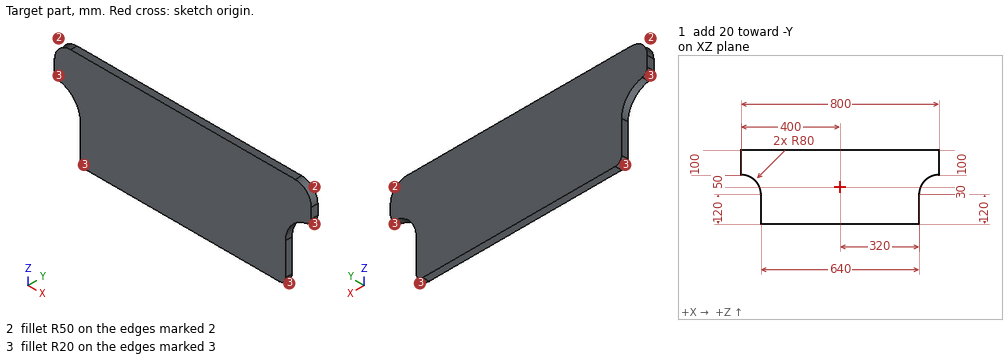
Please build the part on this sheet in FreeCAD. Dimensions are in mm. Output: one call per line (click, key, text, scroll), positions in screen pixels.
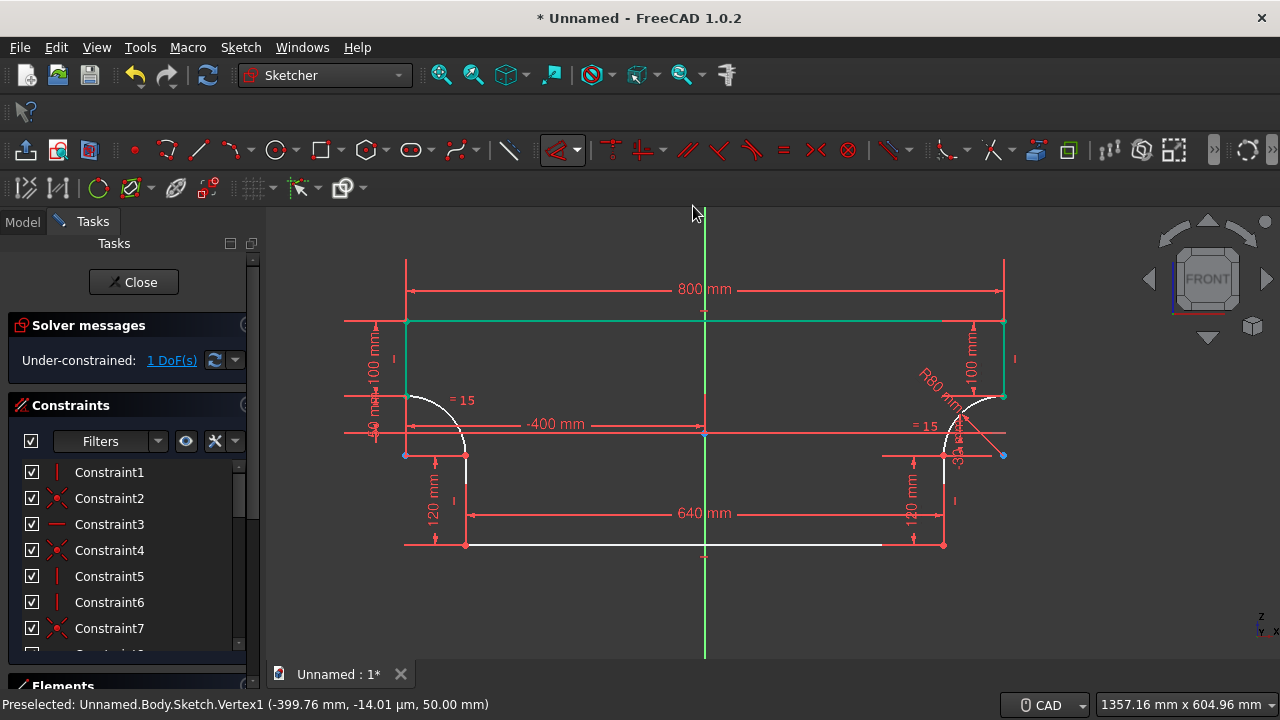
click(944, 456)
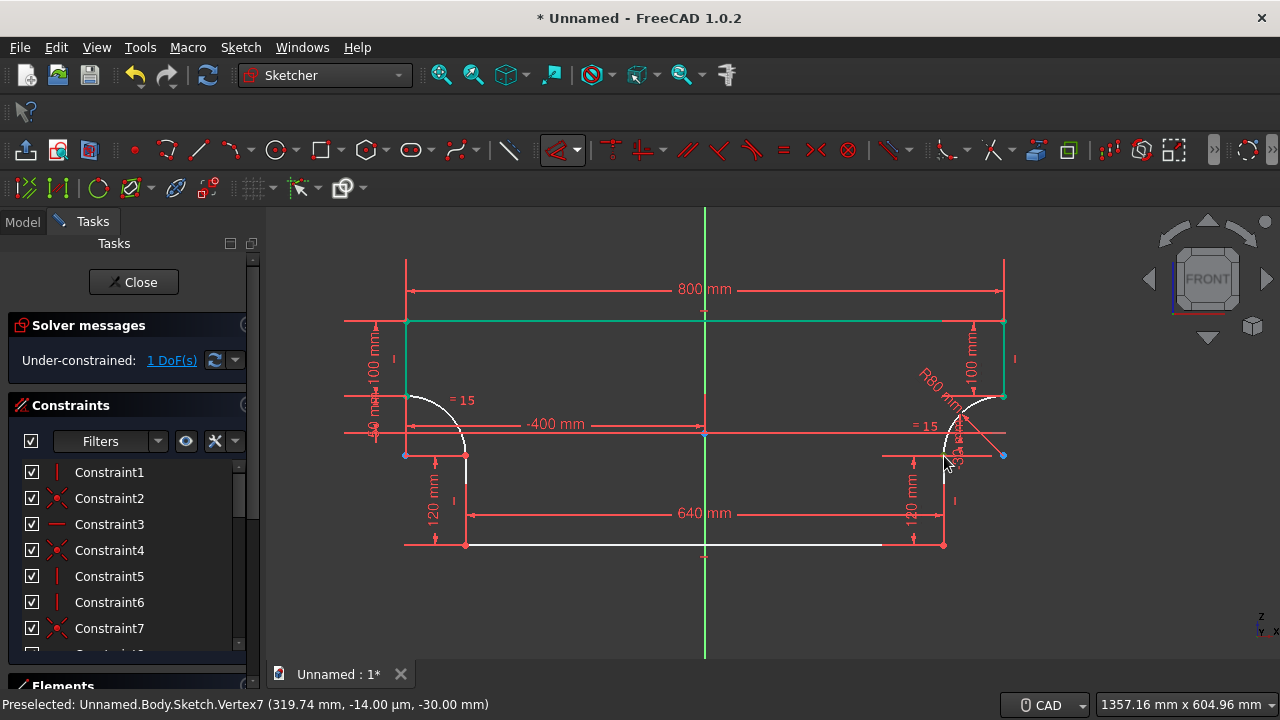
key(l)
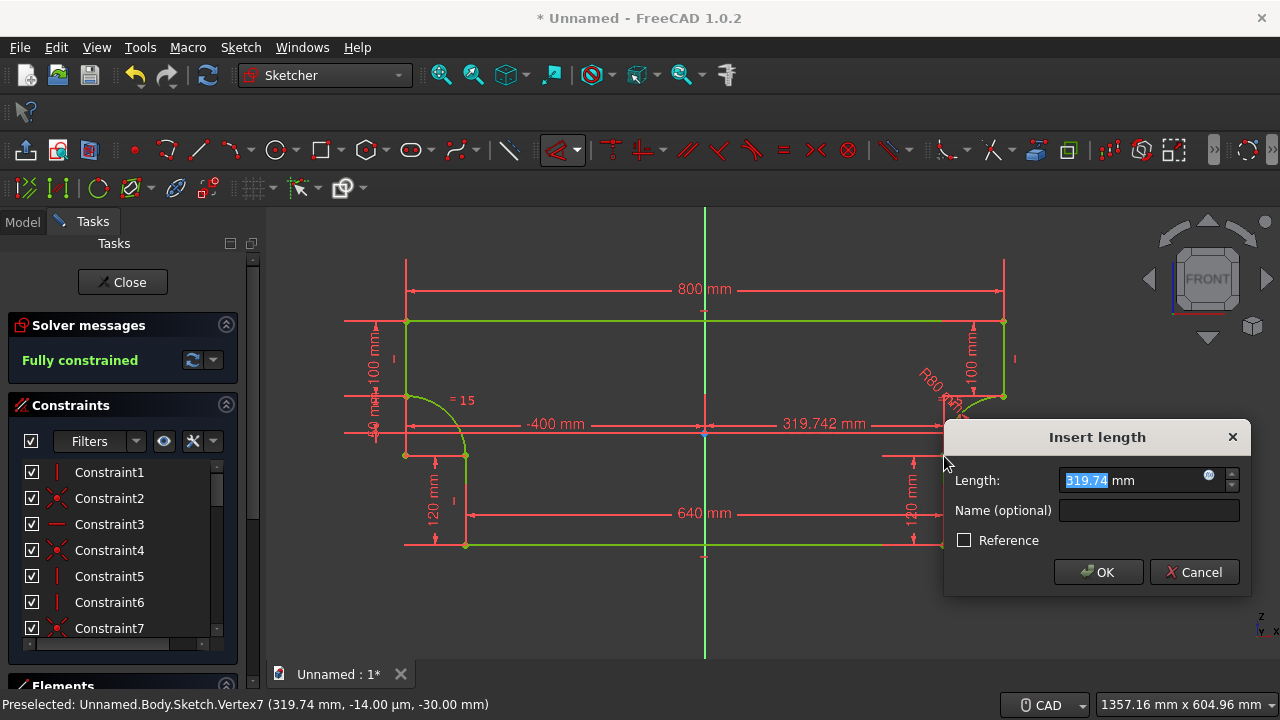
text(320)
key(Return)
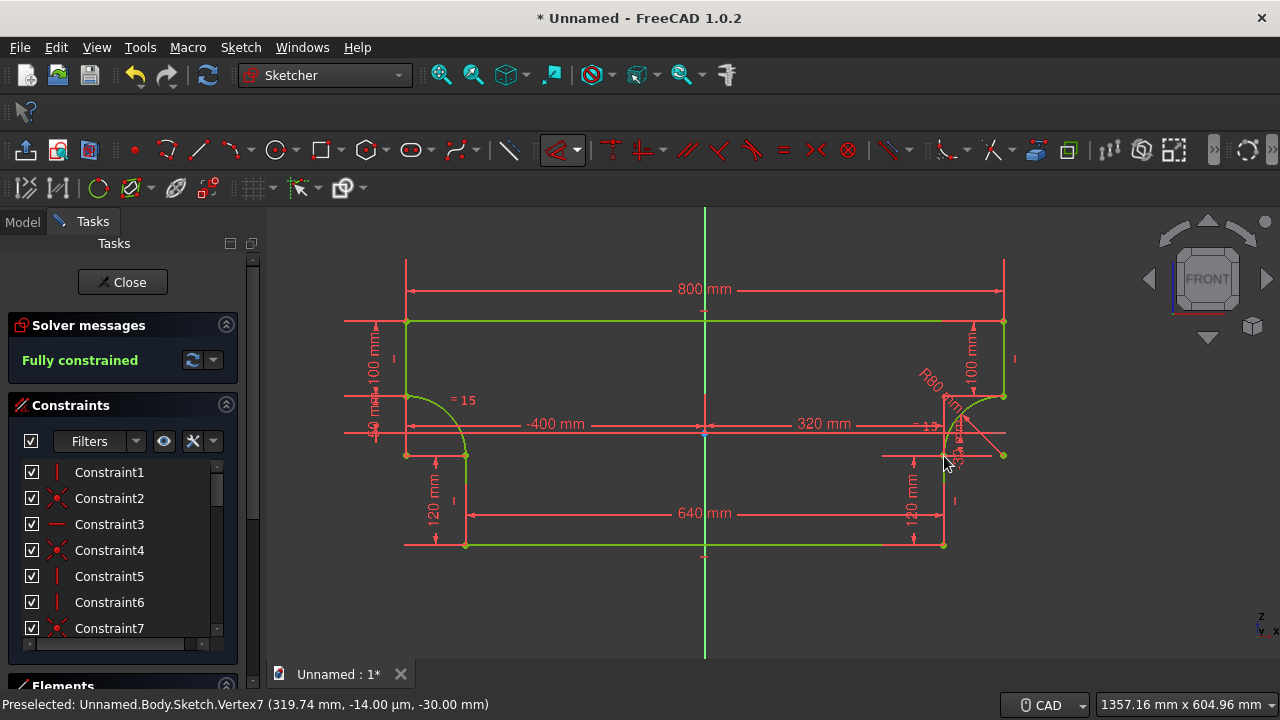
click(123, 282)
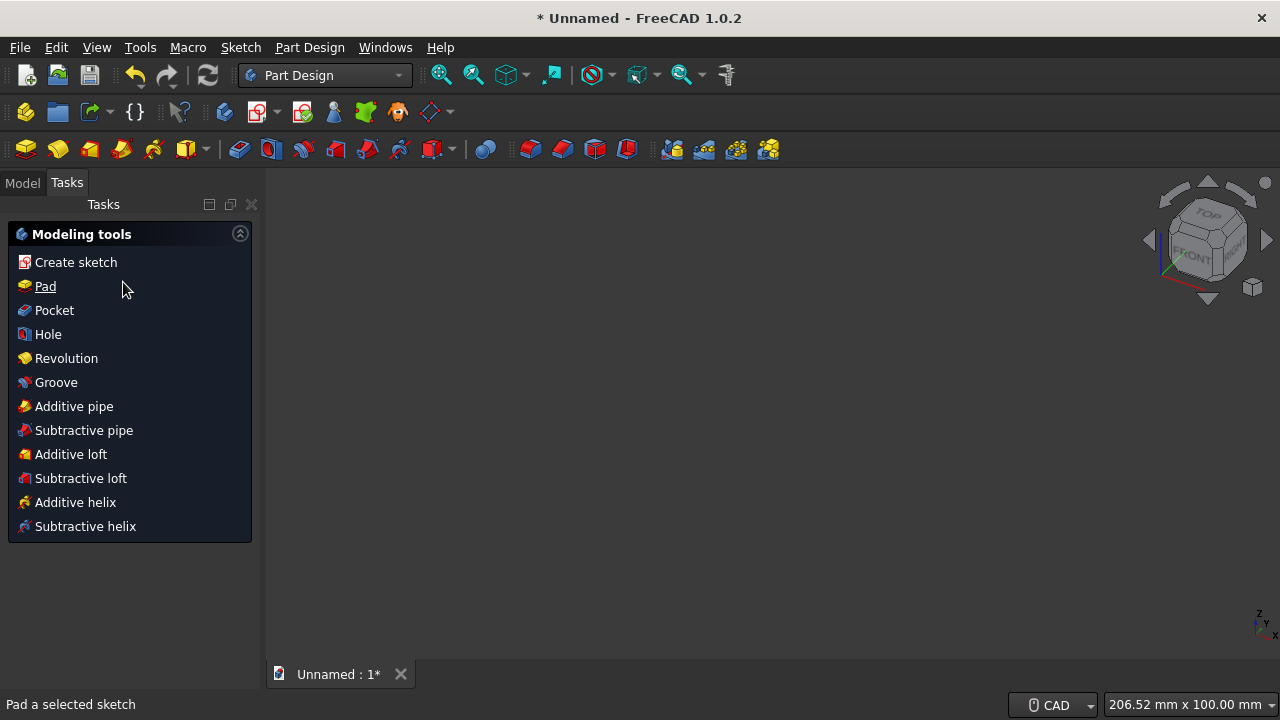
click(26, 150)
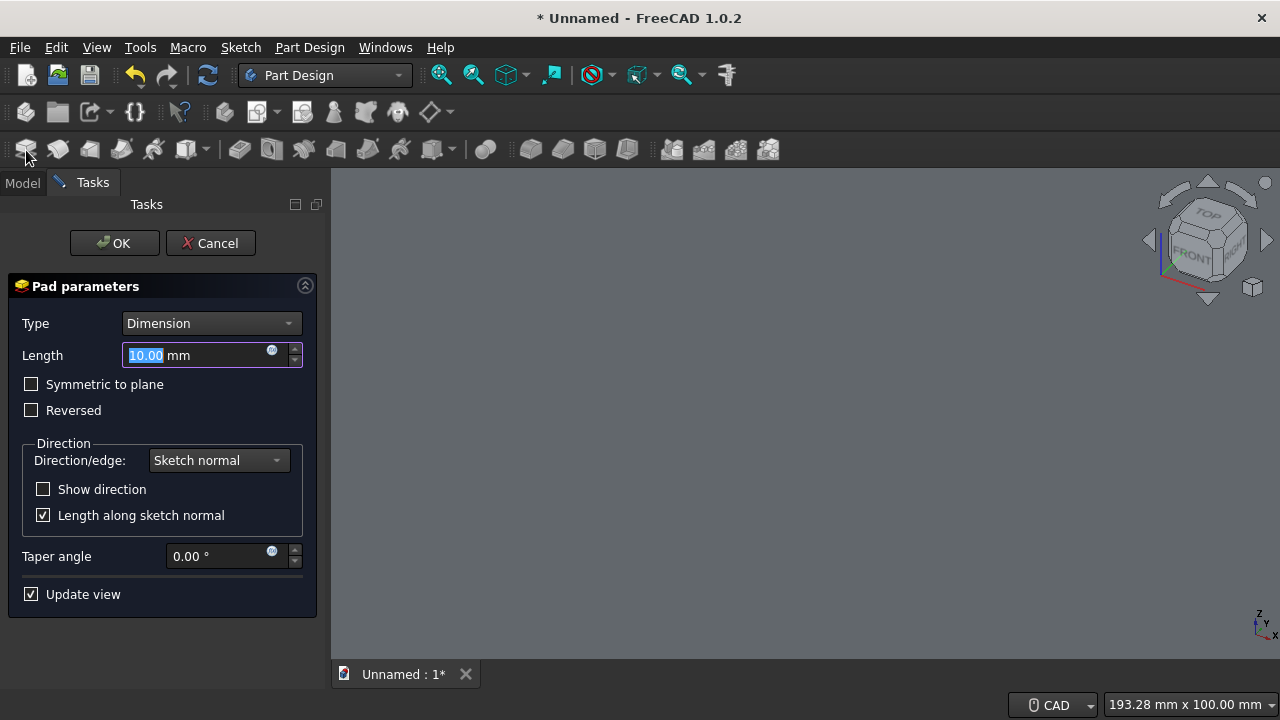
text(20)
key(Tab)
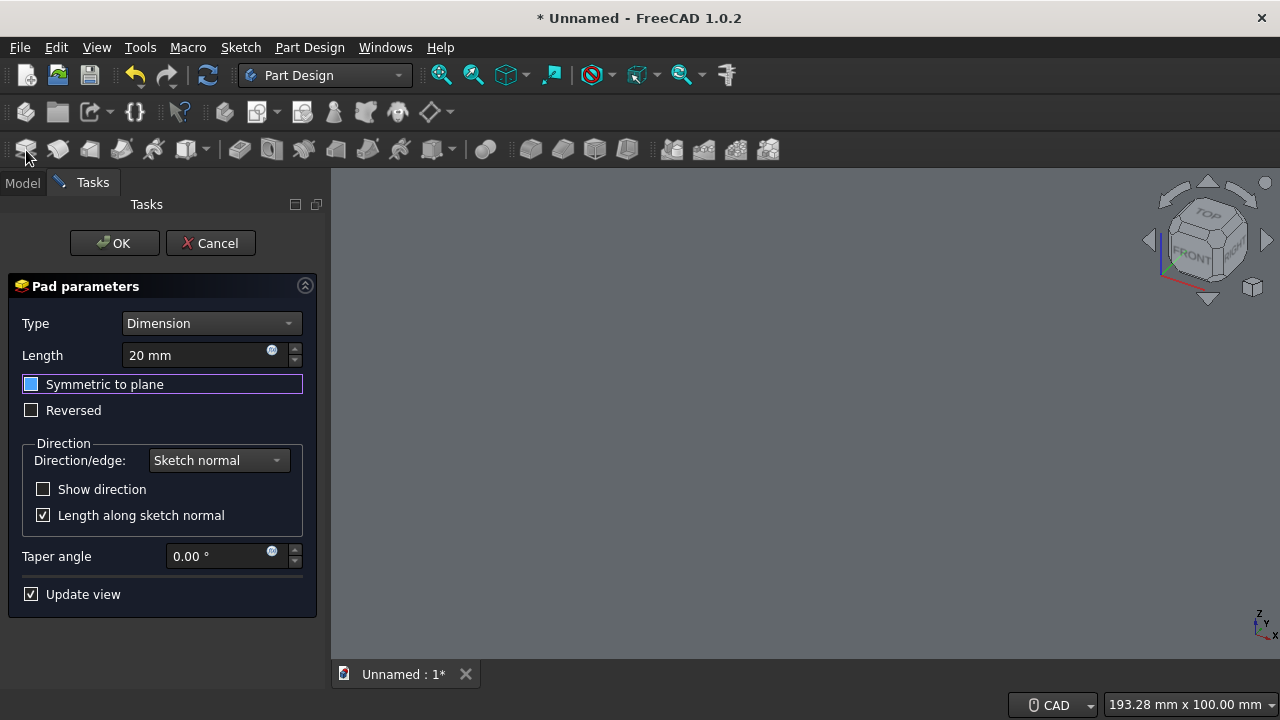
click(115, 243)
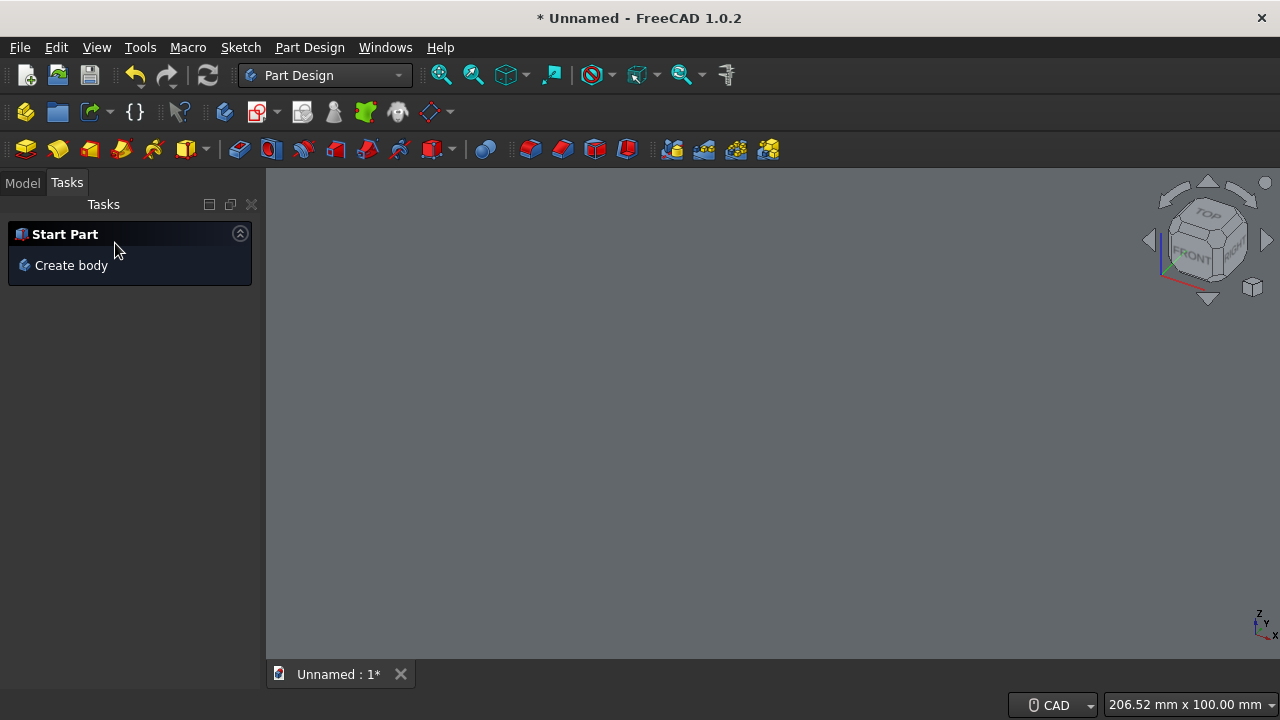
key(v)
key(f)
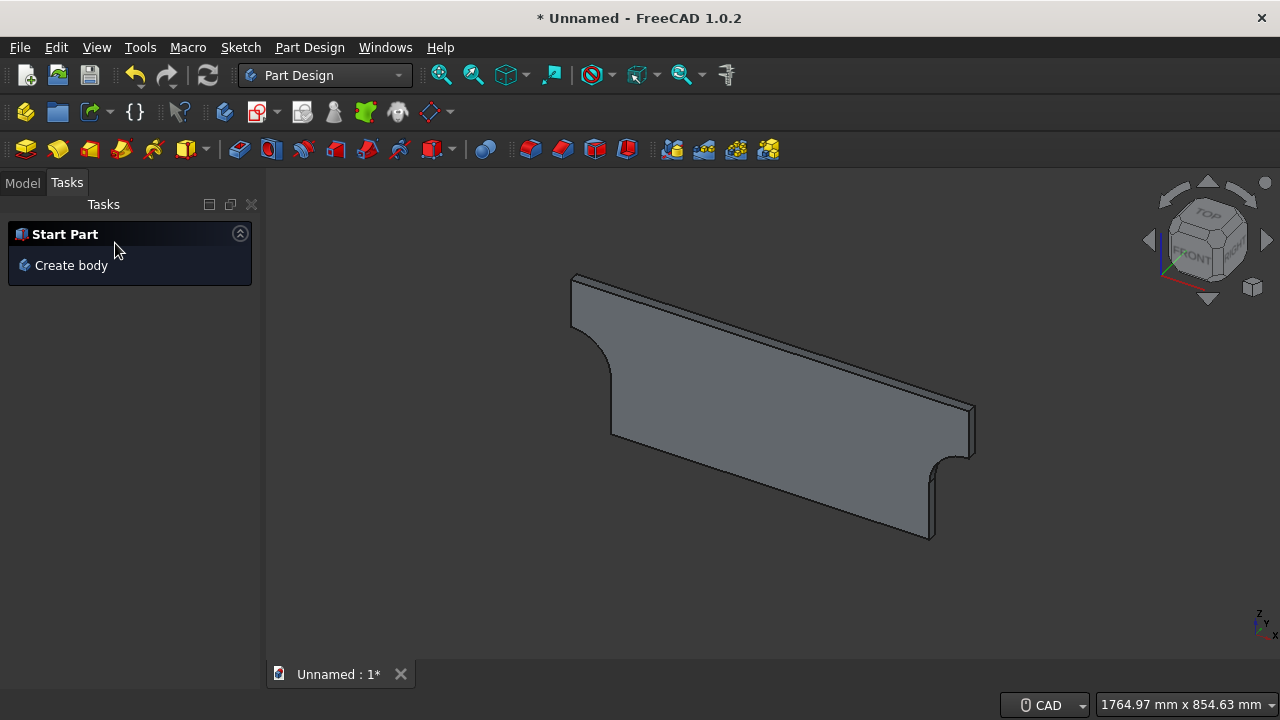
scroll(972, 408, up, 7)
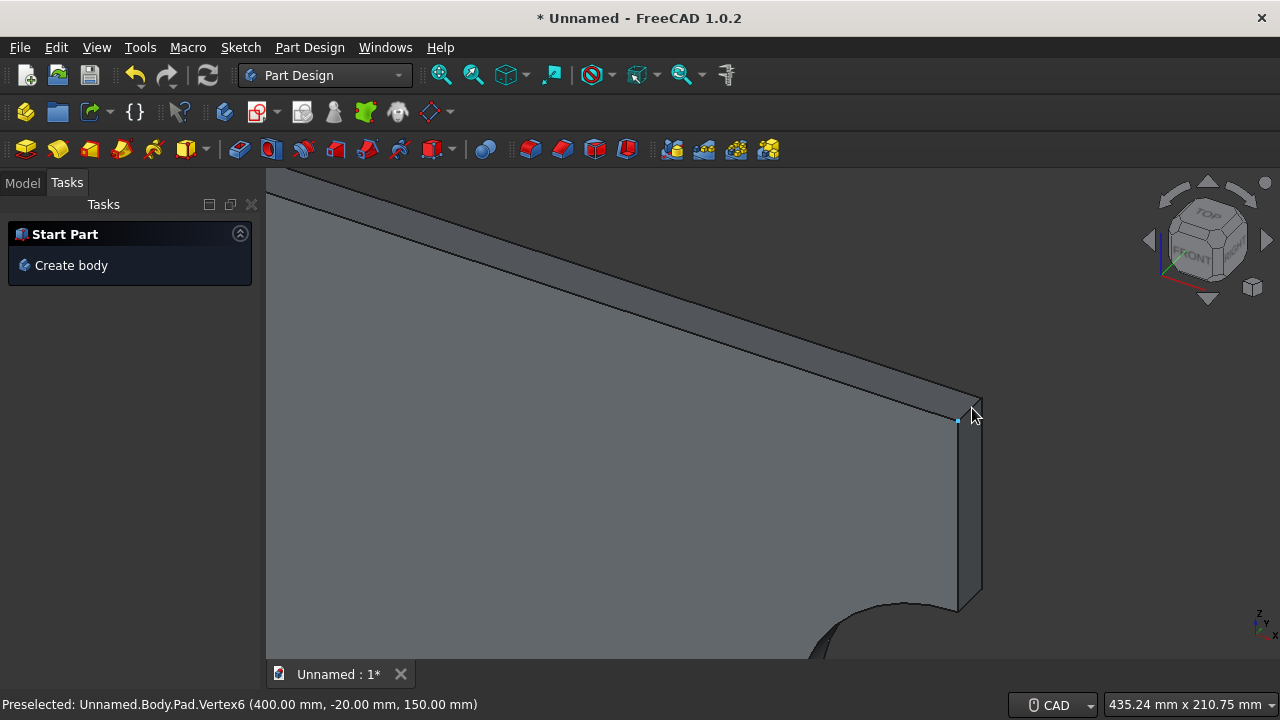
click(970, 409)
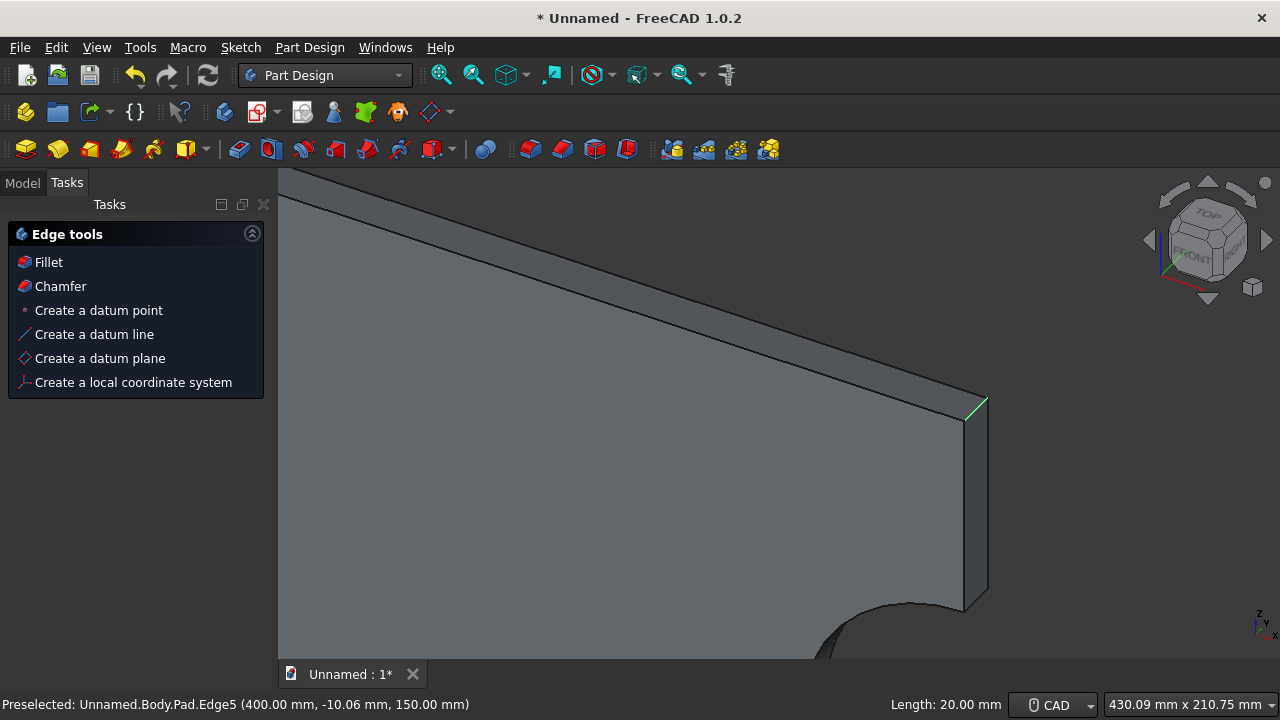
click(442, 76)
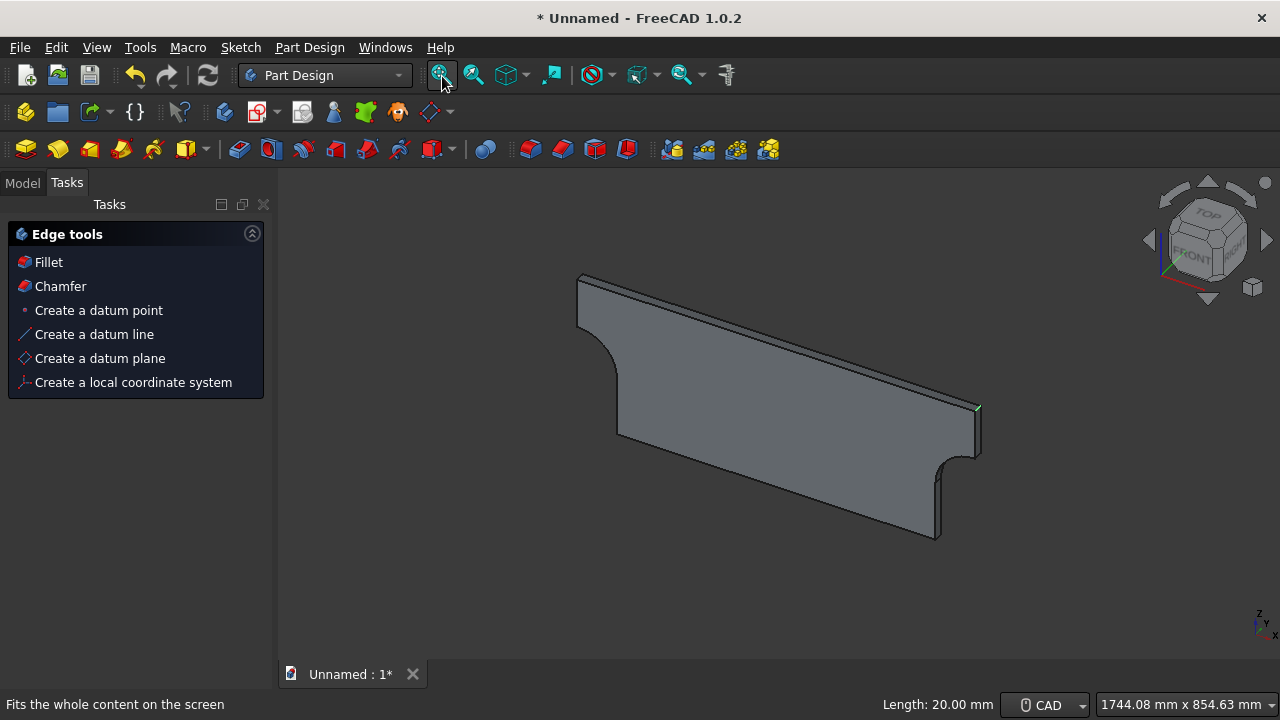
key(0)